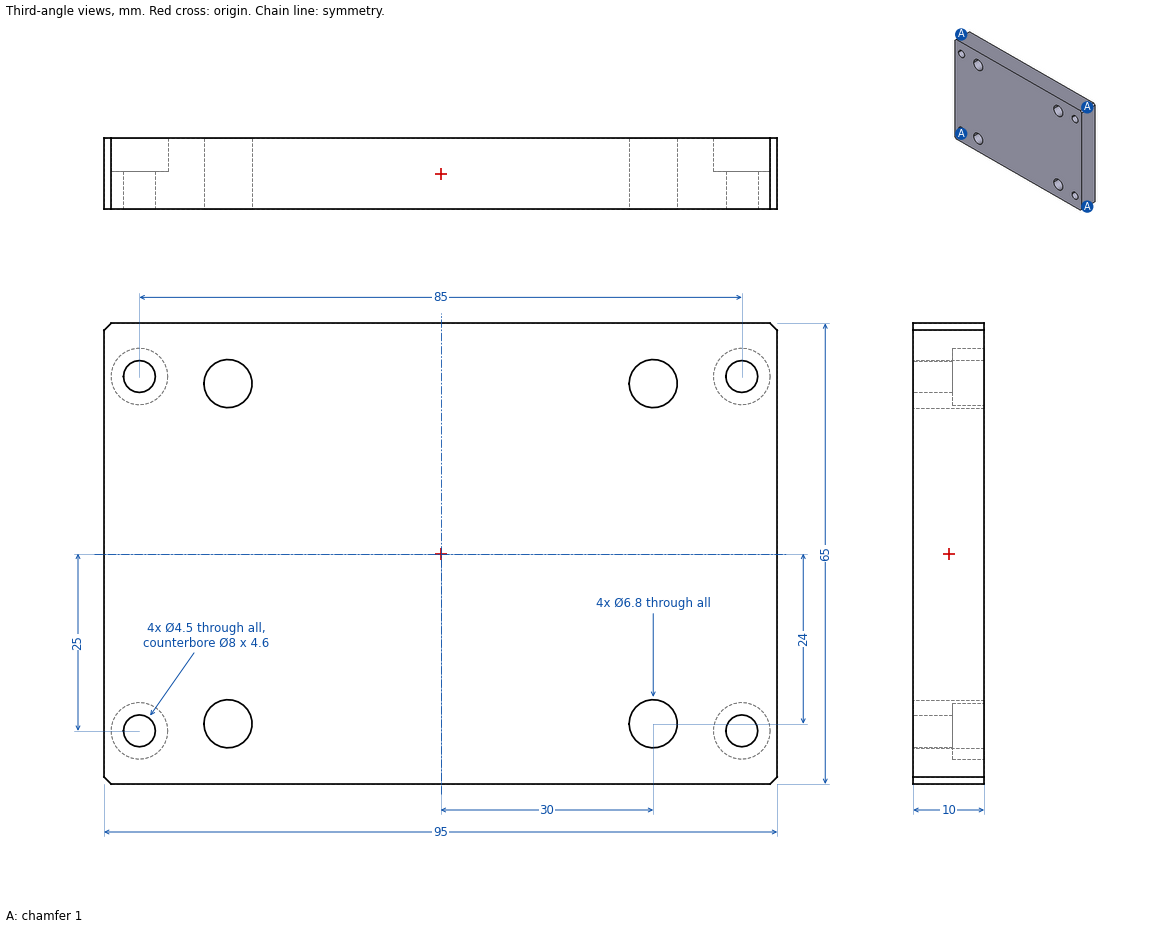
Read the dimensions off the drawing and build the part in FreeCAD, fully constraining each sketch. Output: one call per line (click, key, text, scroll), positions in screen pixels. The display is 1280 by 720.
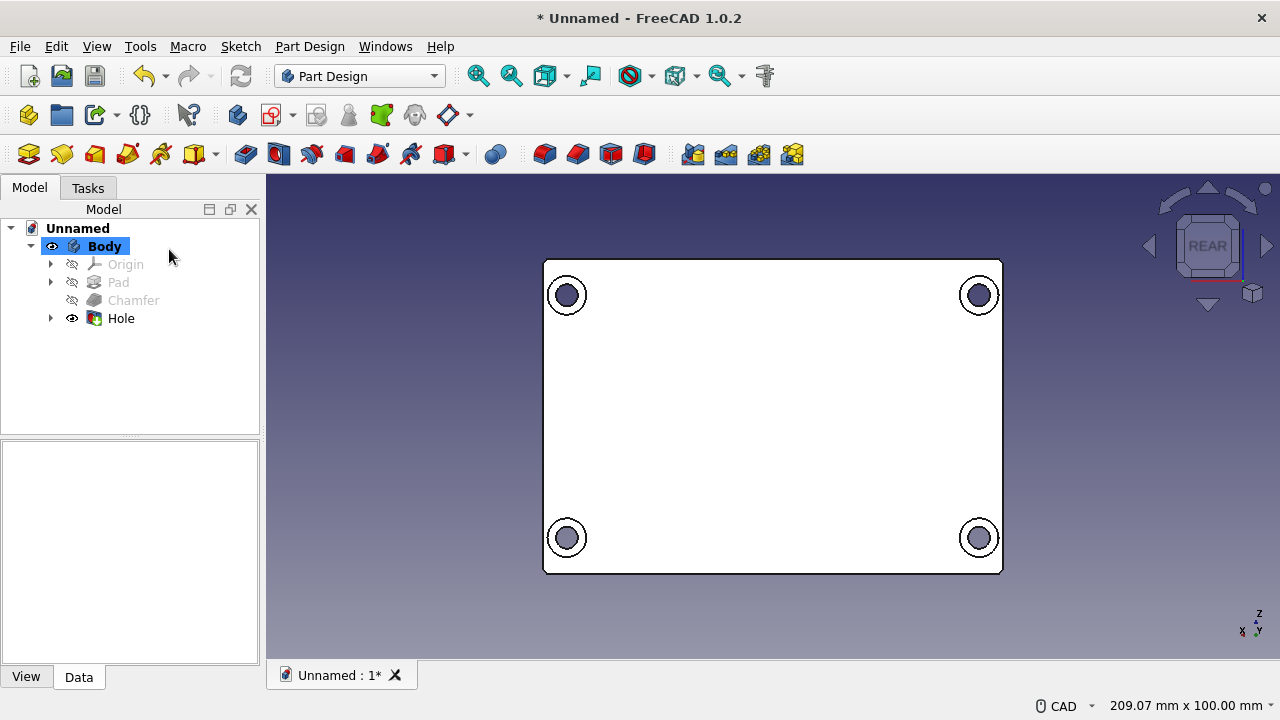
click(707, 415)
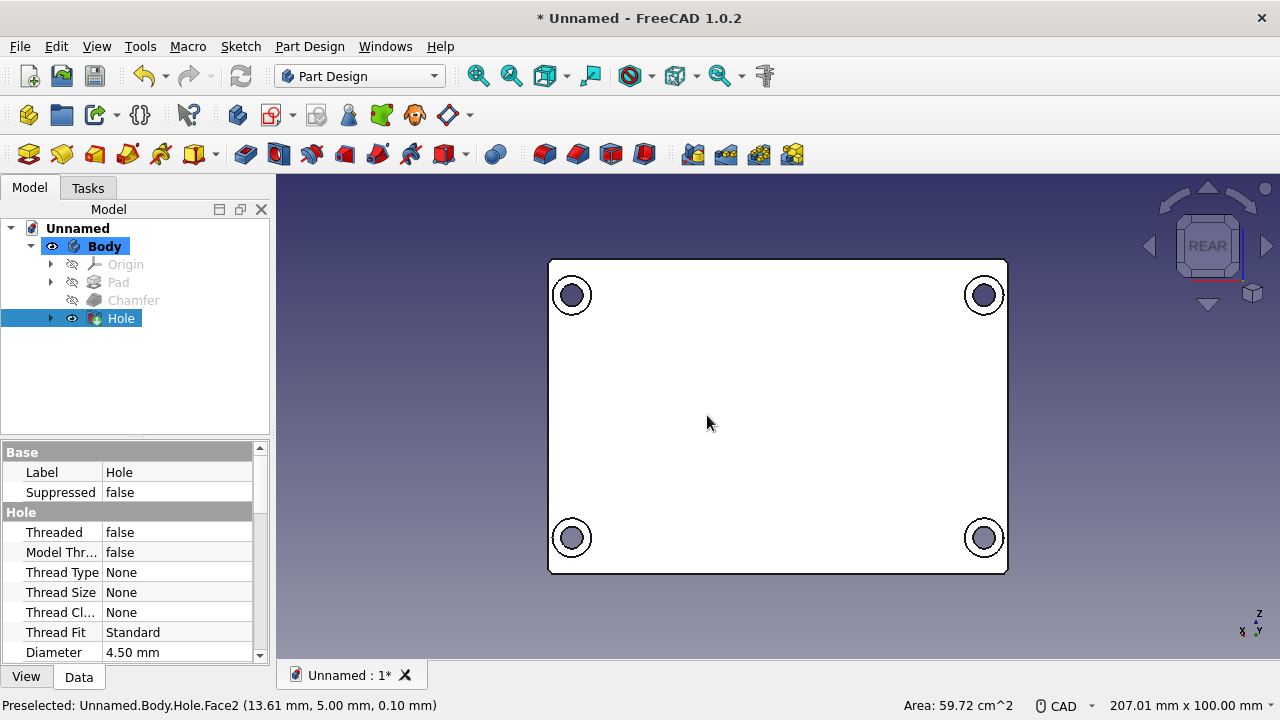
click(270, 116)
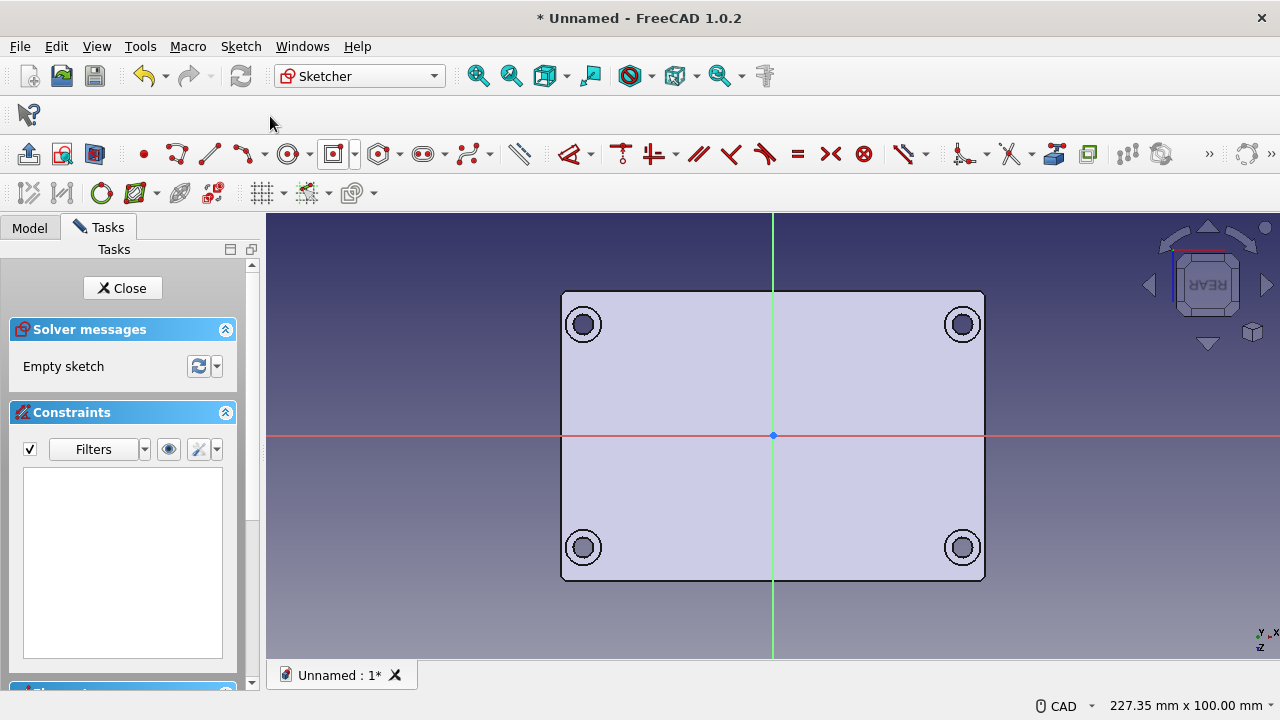
click(288, 154)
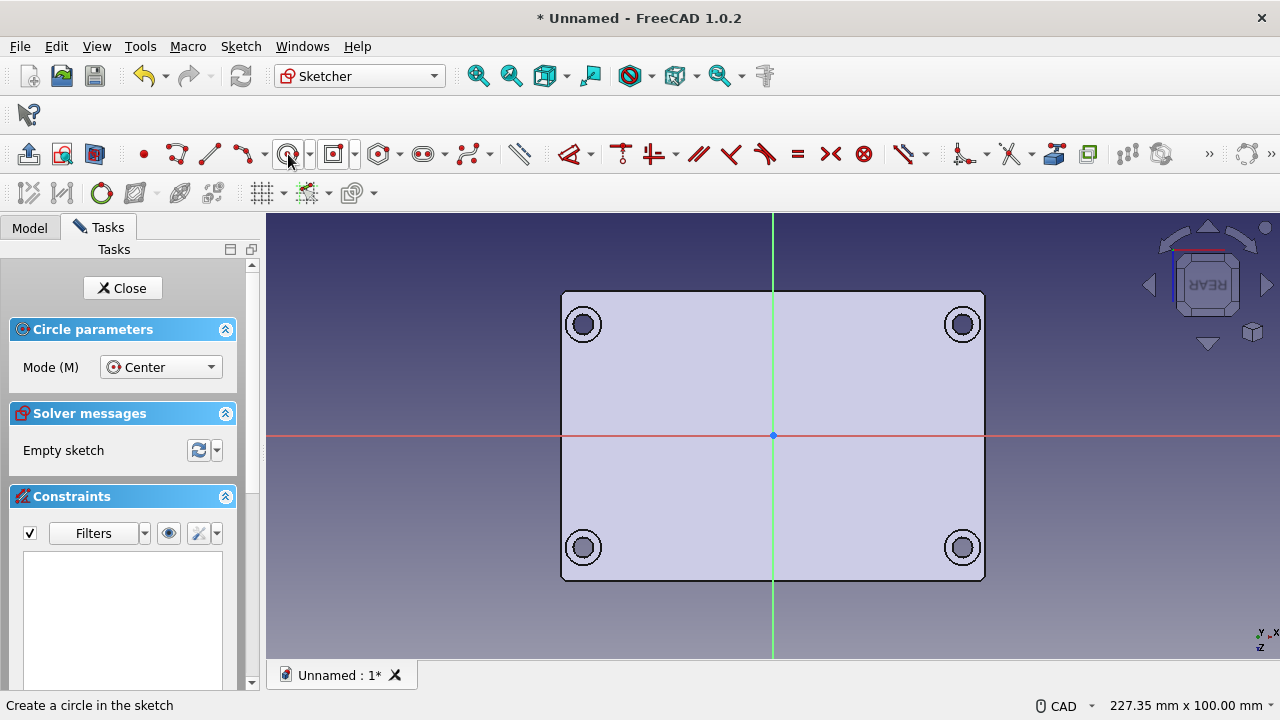
scroll(907, 329, up, 3)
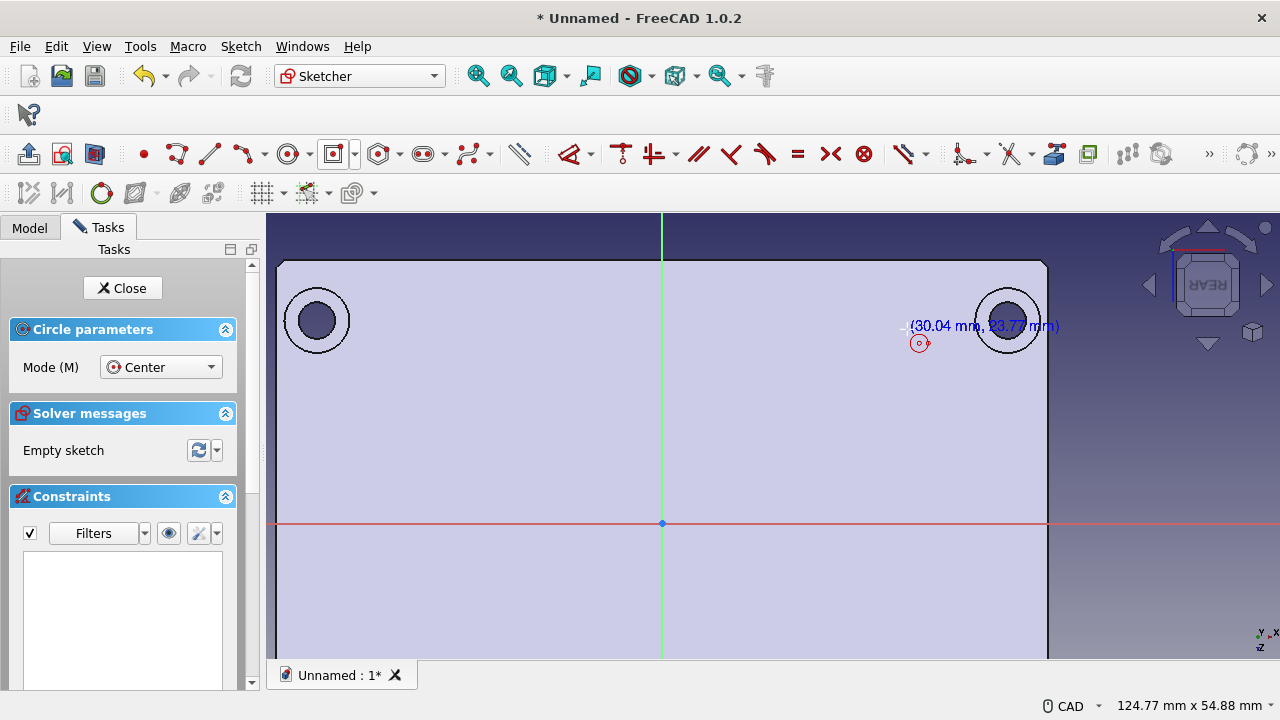
click(906, 329)
move(926, 309)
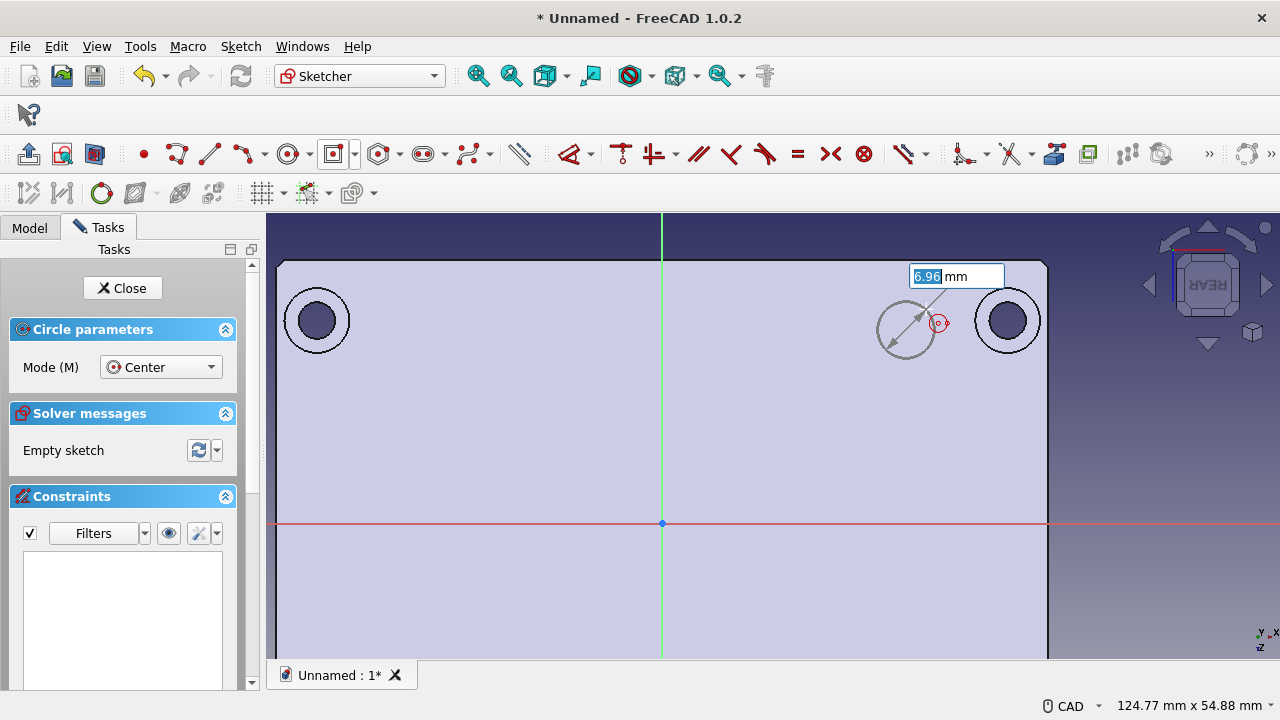
text(6.8)
key(Return)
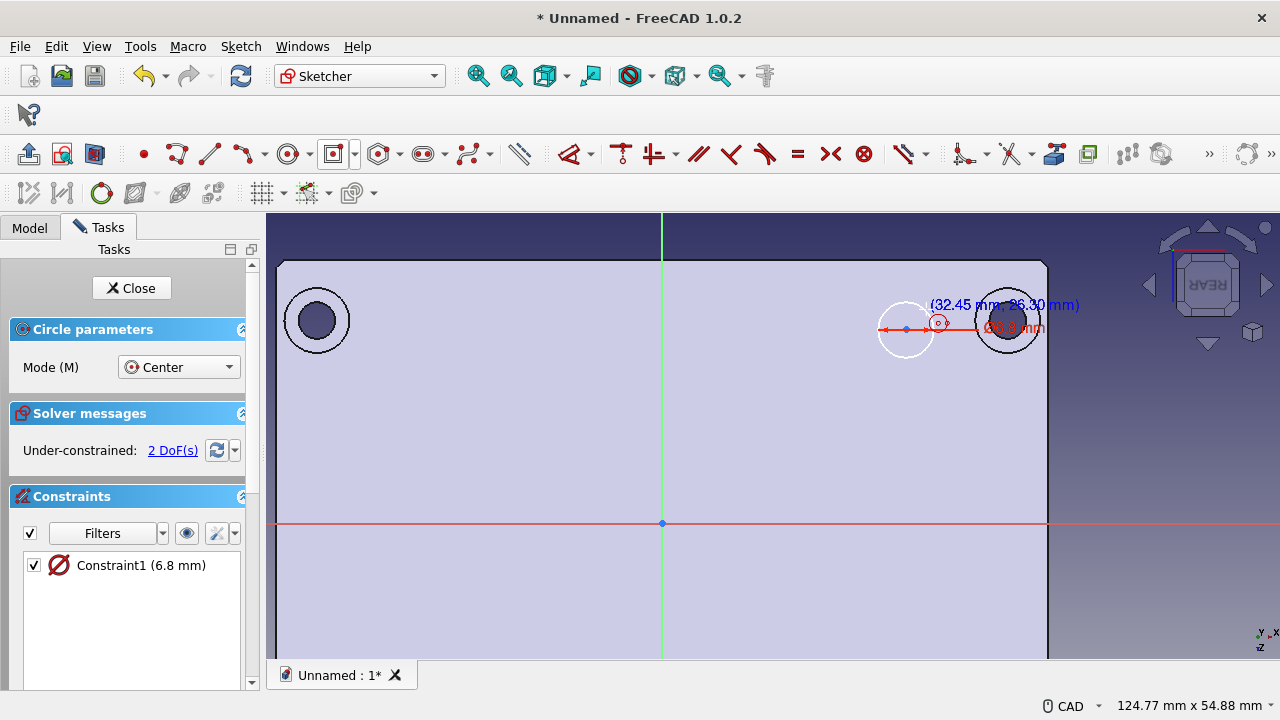
scroll(790, 258, down, 2)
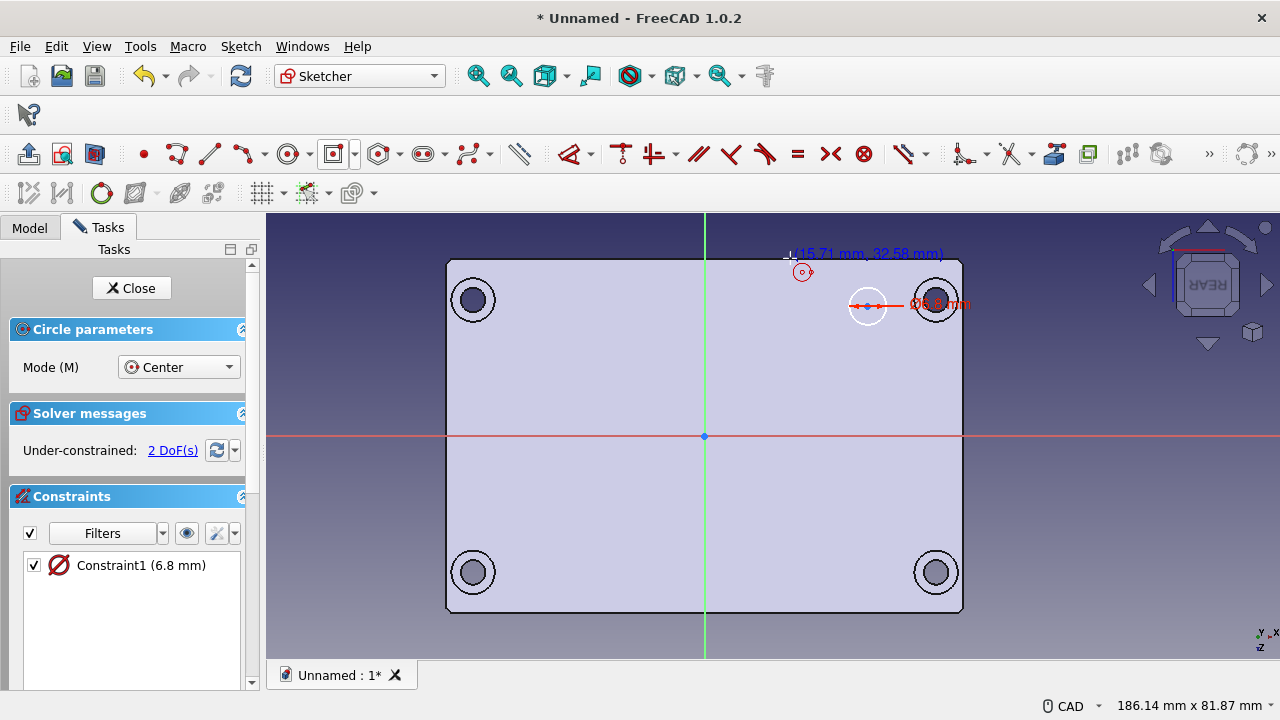
scroll(868, 567, up, 2)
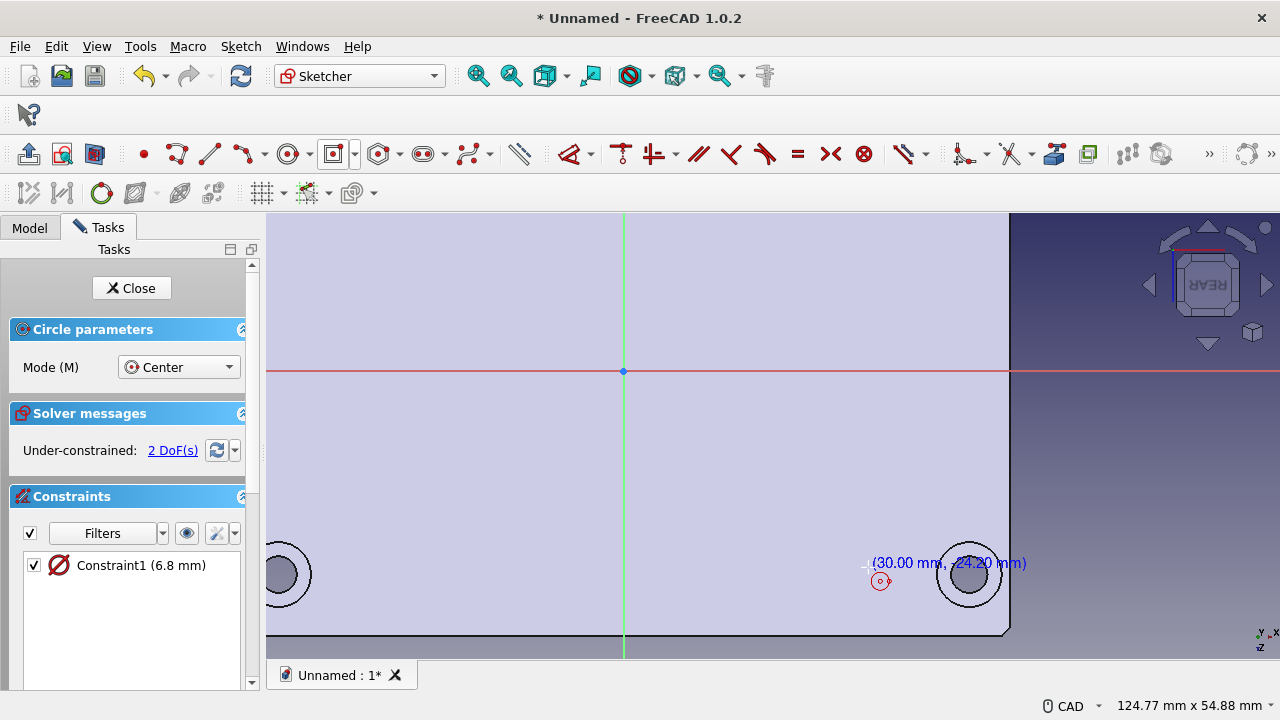
click(868, 566)
move(887, 547)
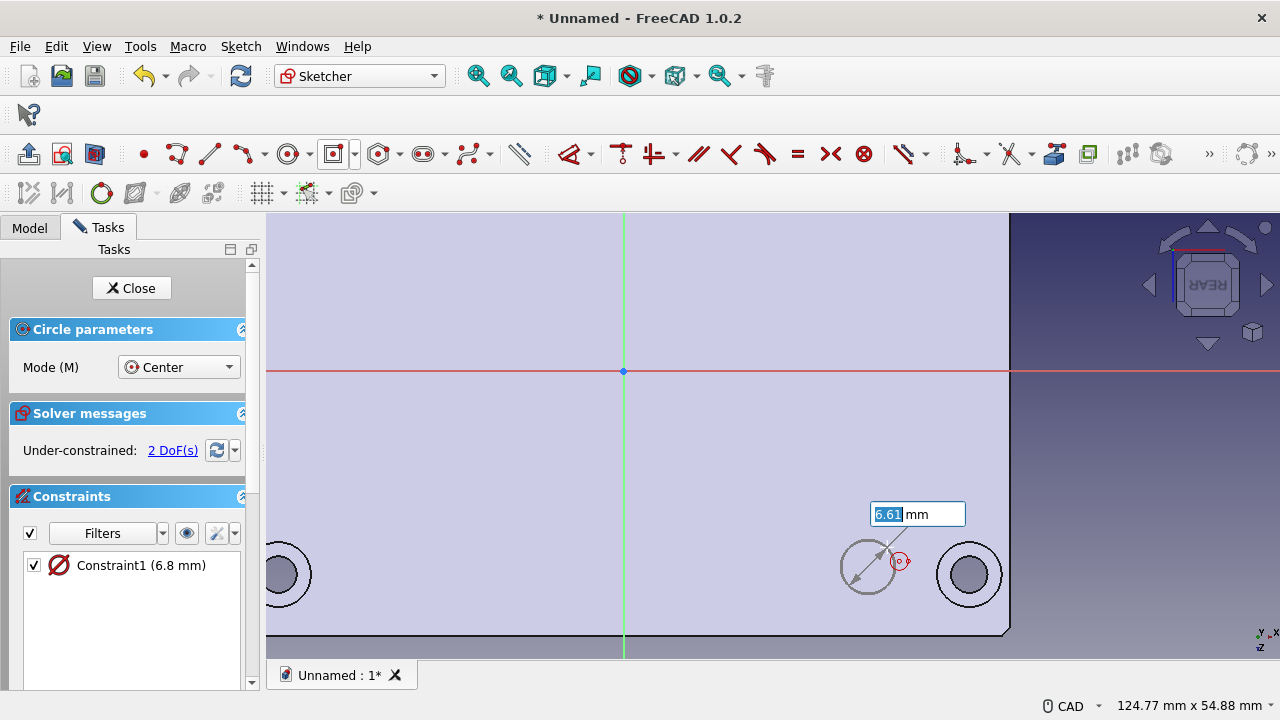
text(6.8)
key(Return)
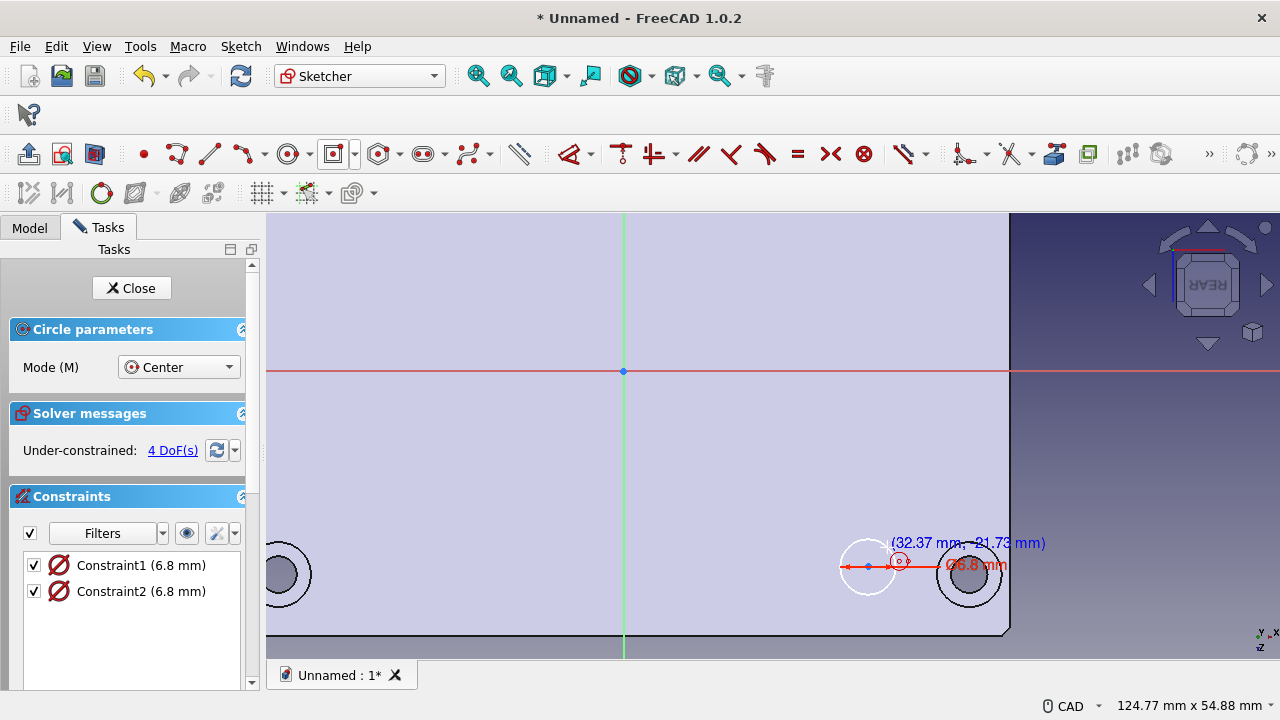
click(380, 566)
move(400, 547)